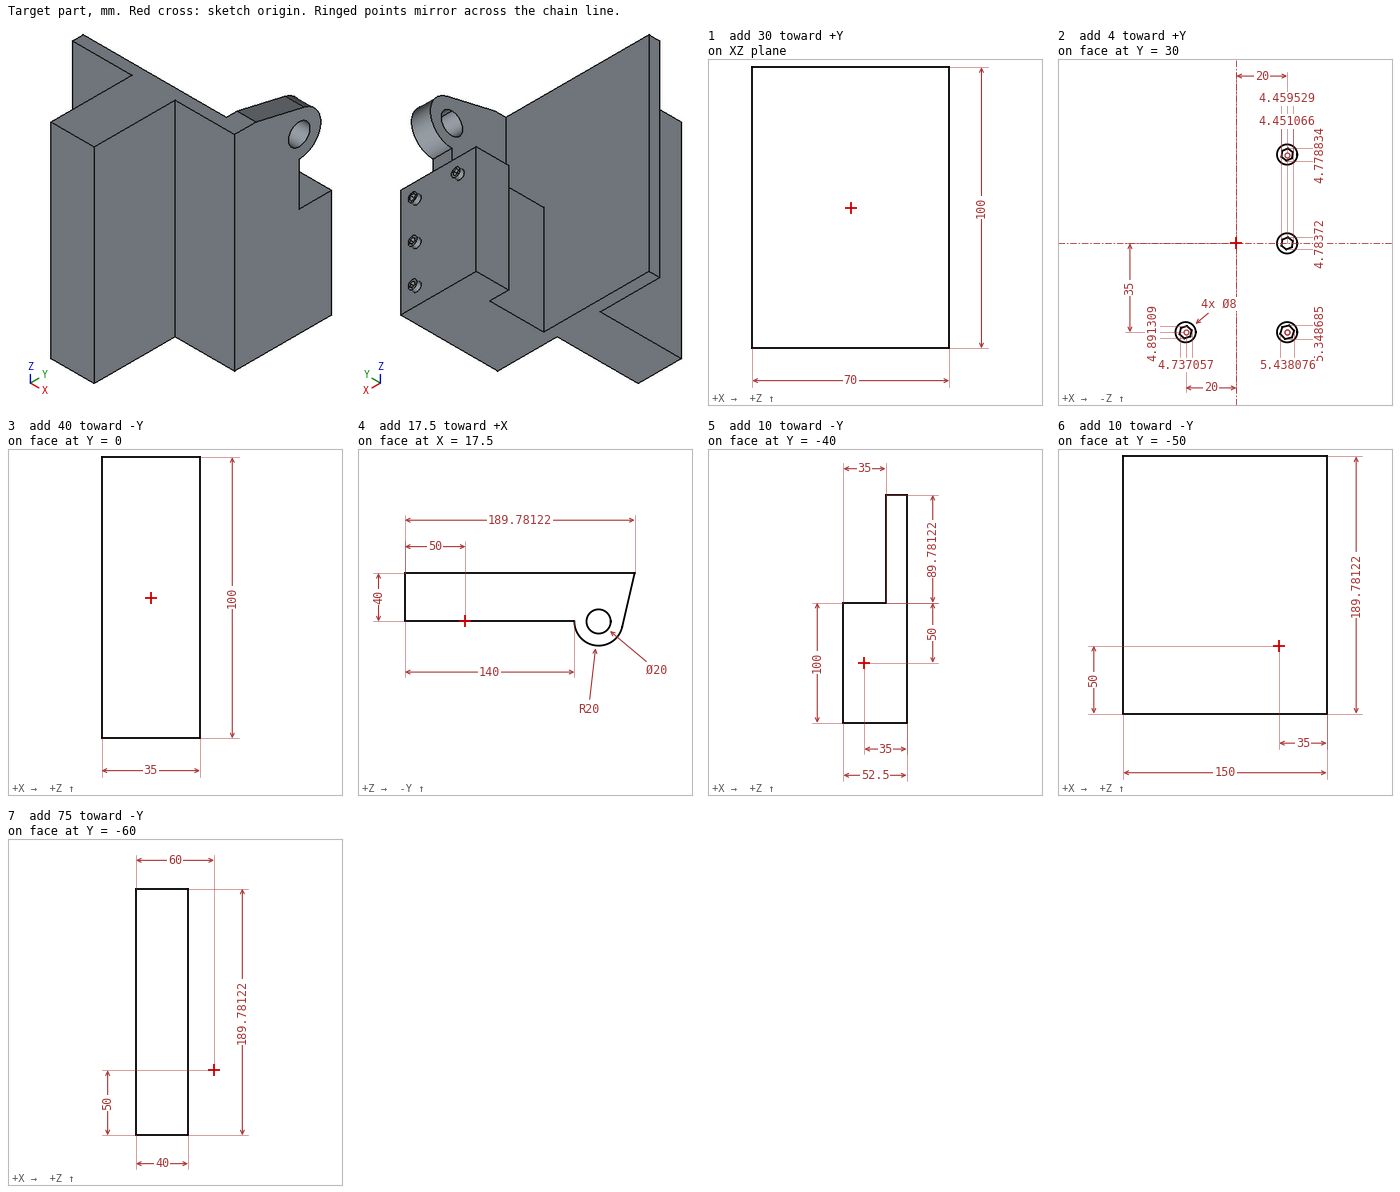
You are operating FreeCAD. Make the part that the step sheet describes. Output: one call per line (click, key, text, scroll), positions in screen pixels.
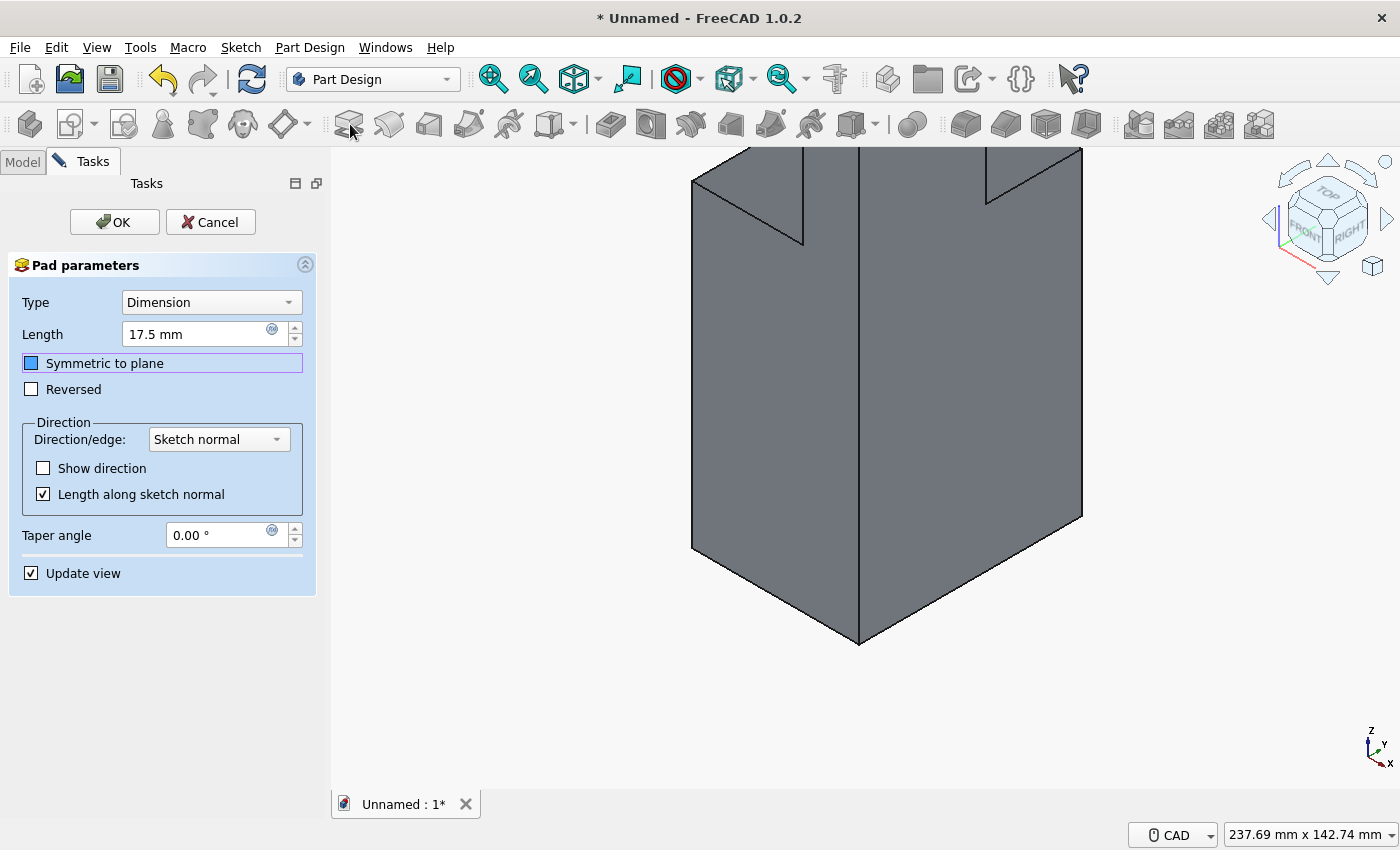
click(115, 222)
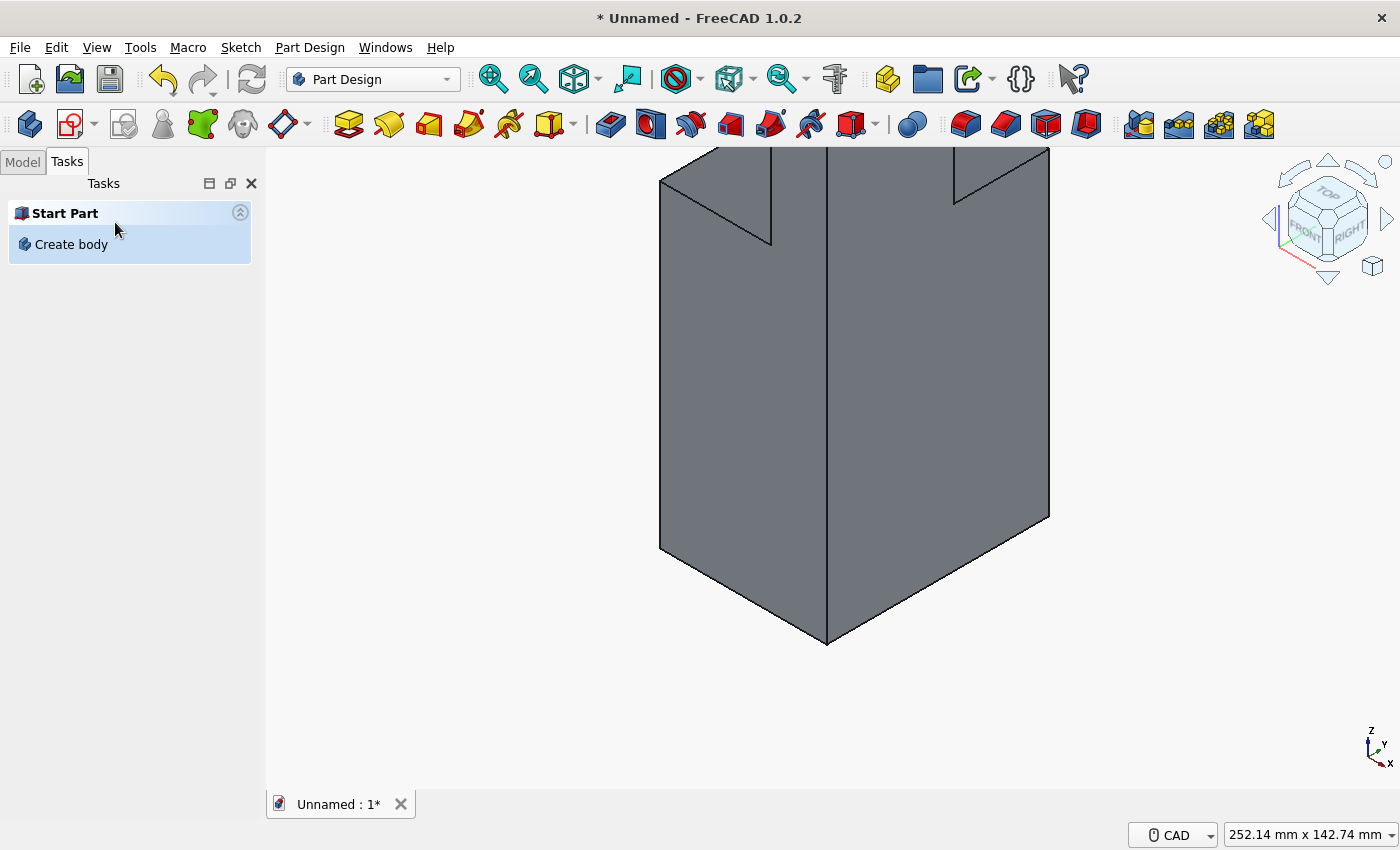
click(494, 80)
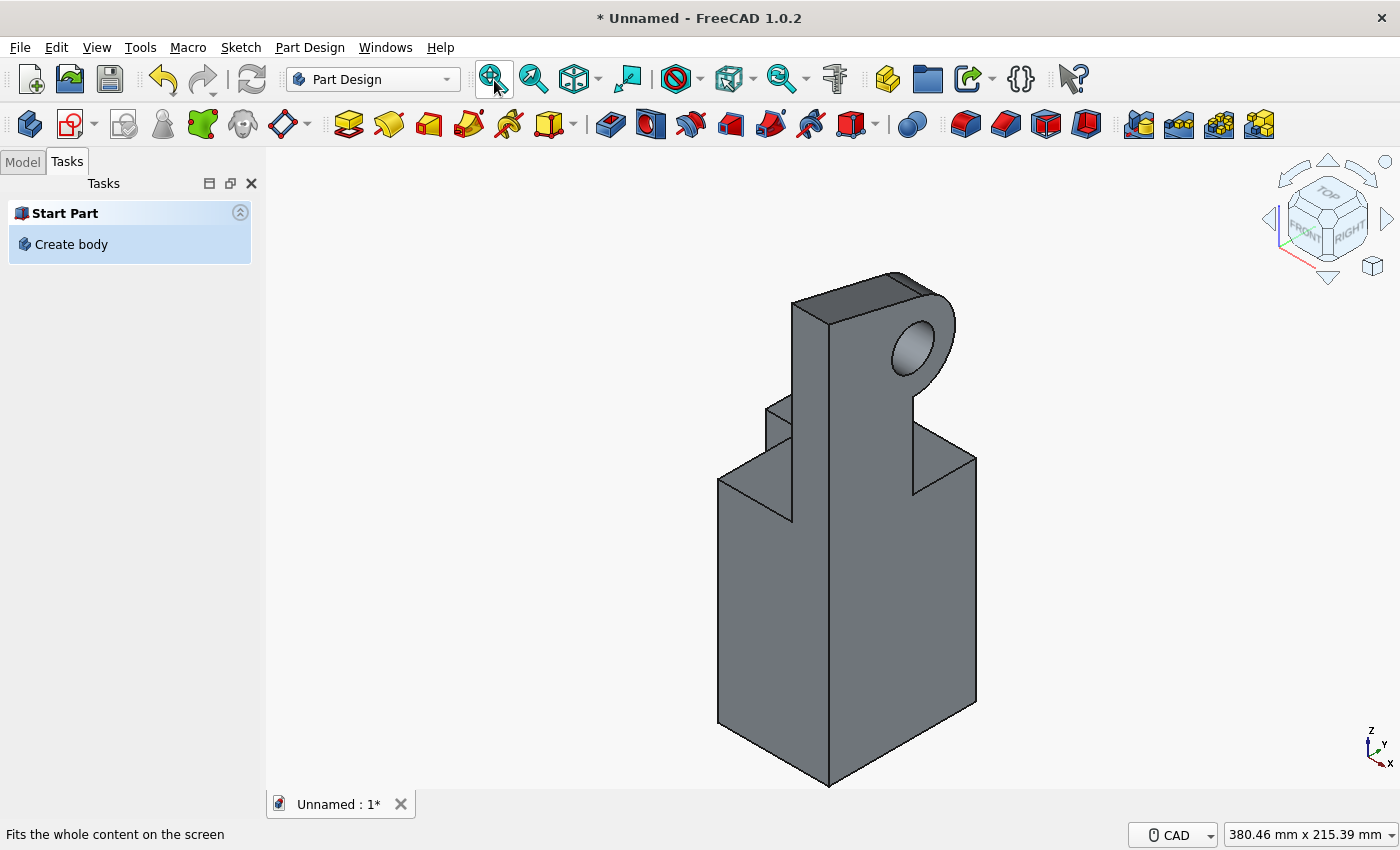
click(773, 589)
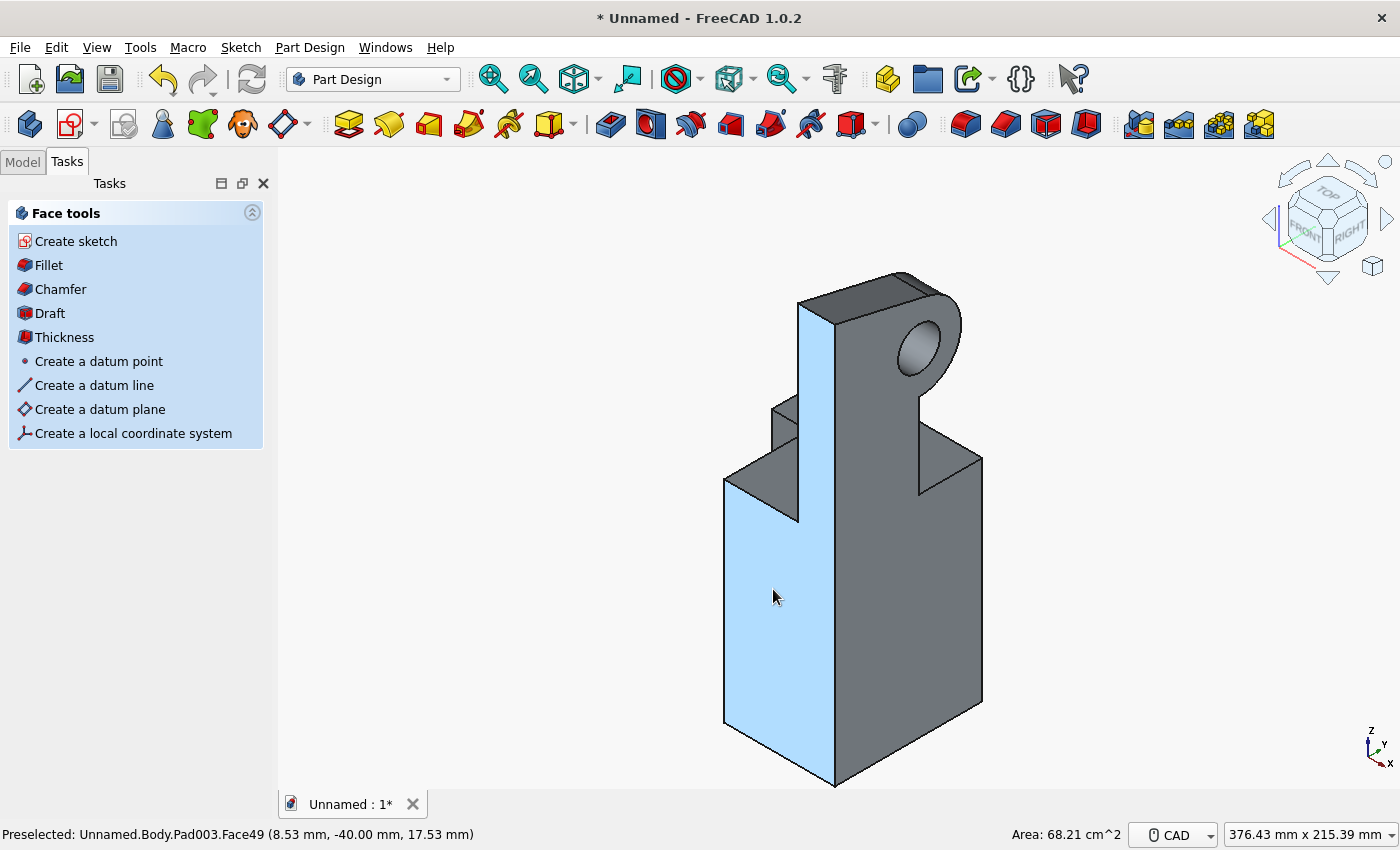
click(70, 124)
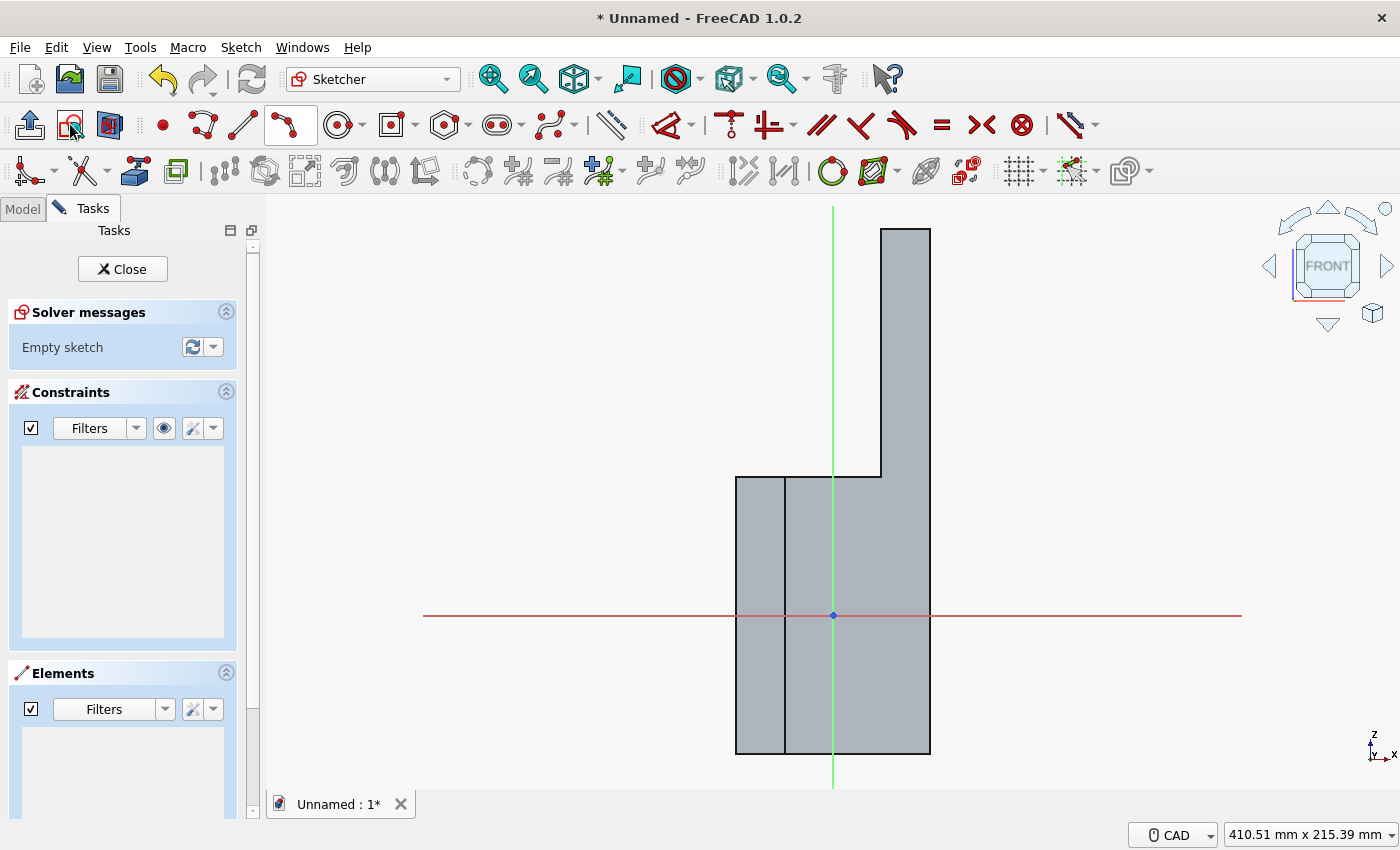
scroll(576, 492, down, 2)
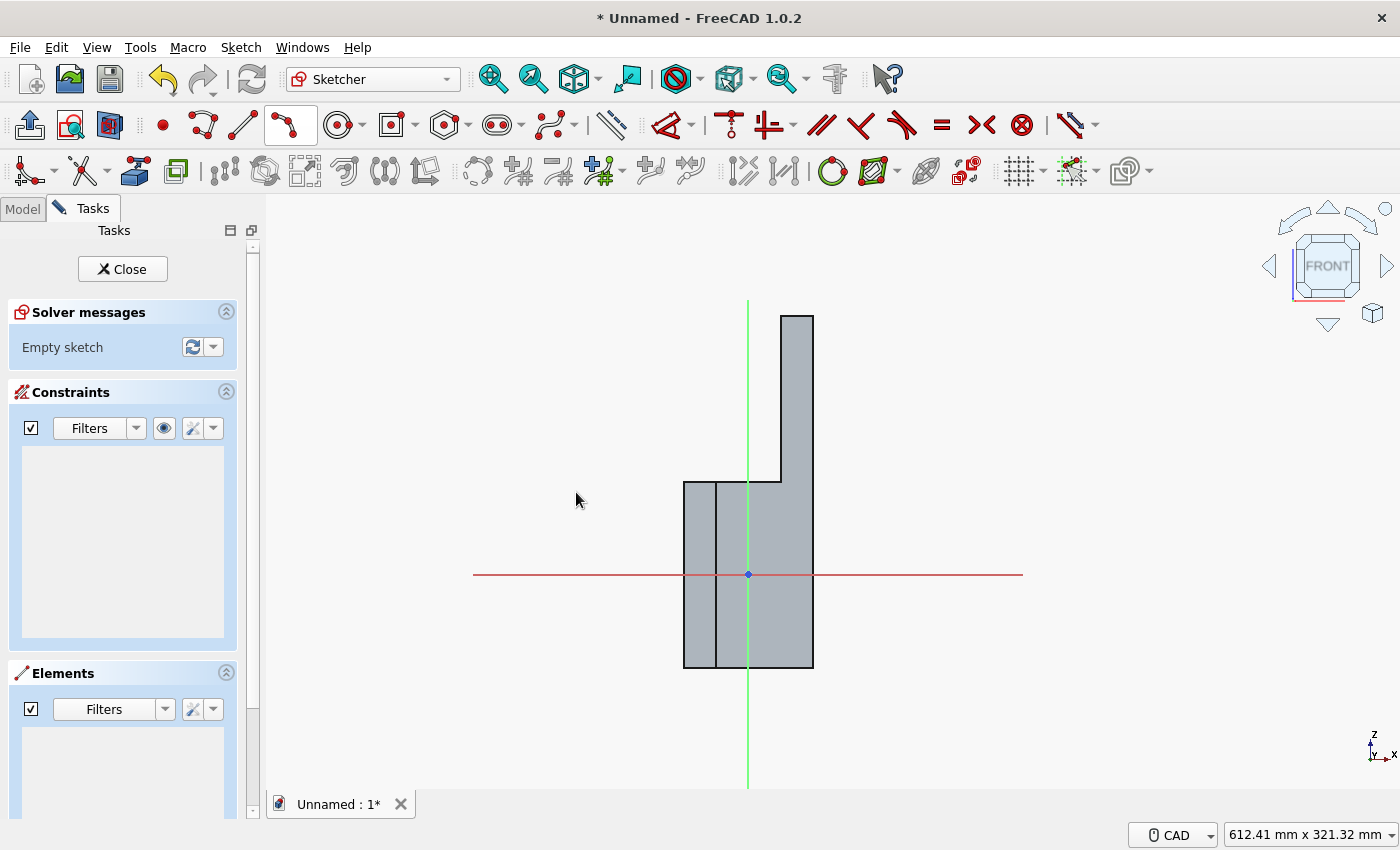
click(204, 126)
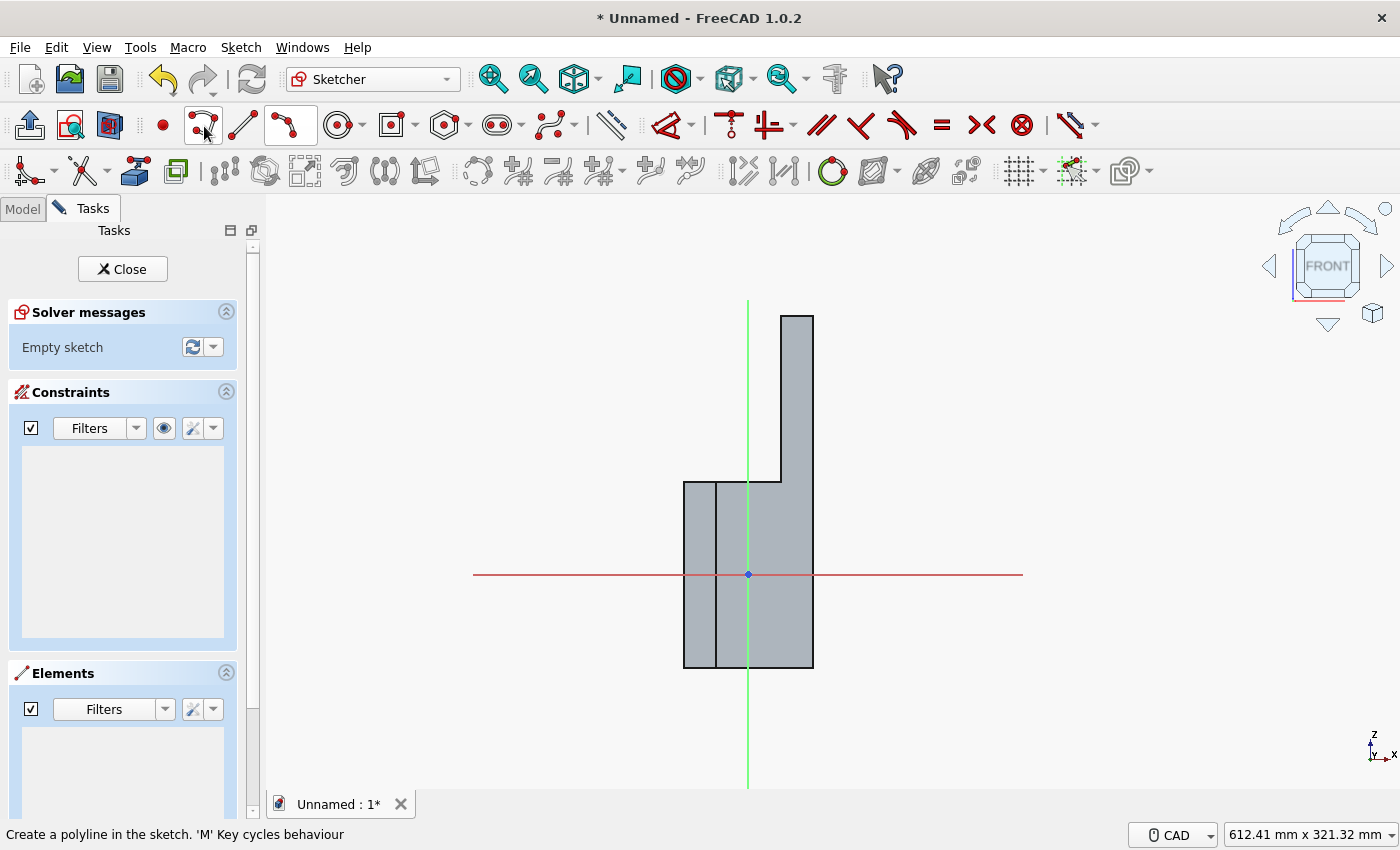
click(781, 482)
click(716, 482)
click(716, 668)
click(813, 668)
click(813, 316)
click(781, 316)
click(781, 483)
key(Escape)
key(Escape)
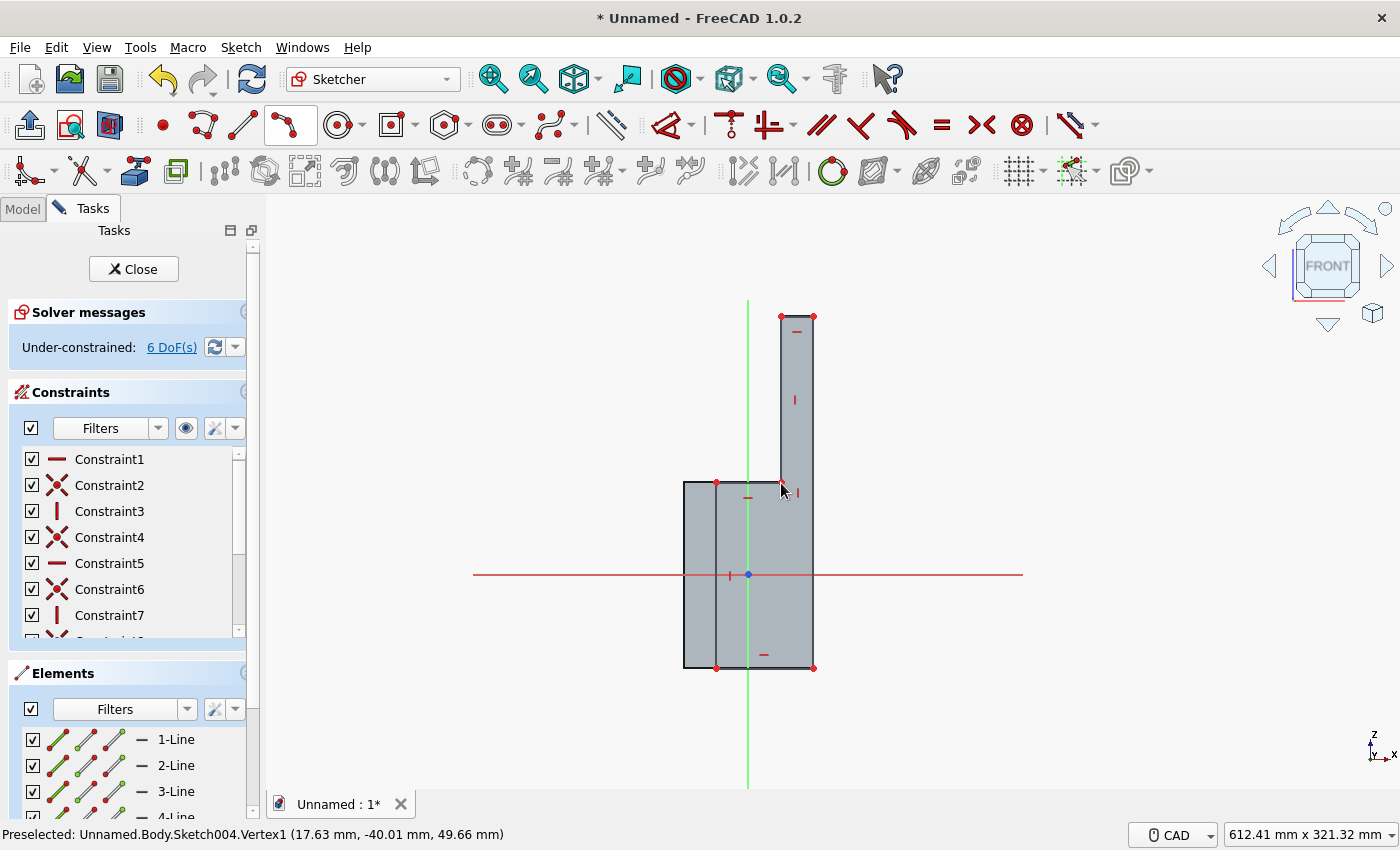
click(666, 126)